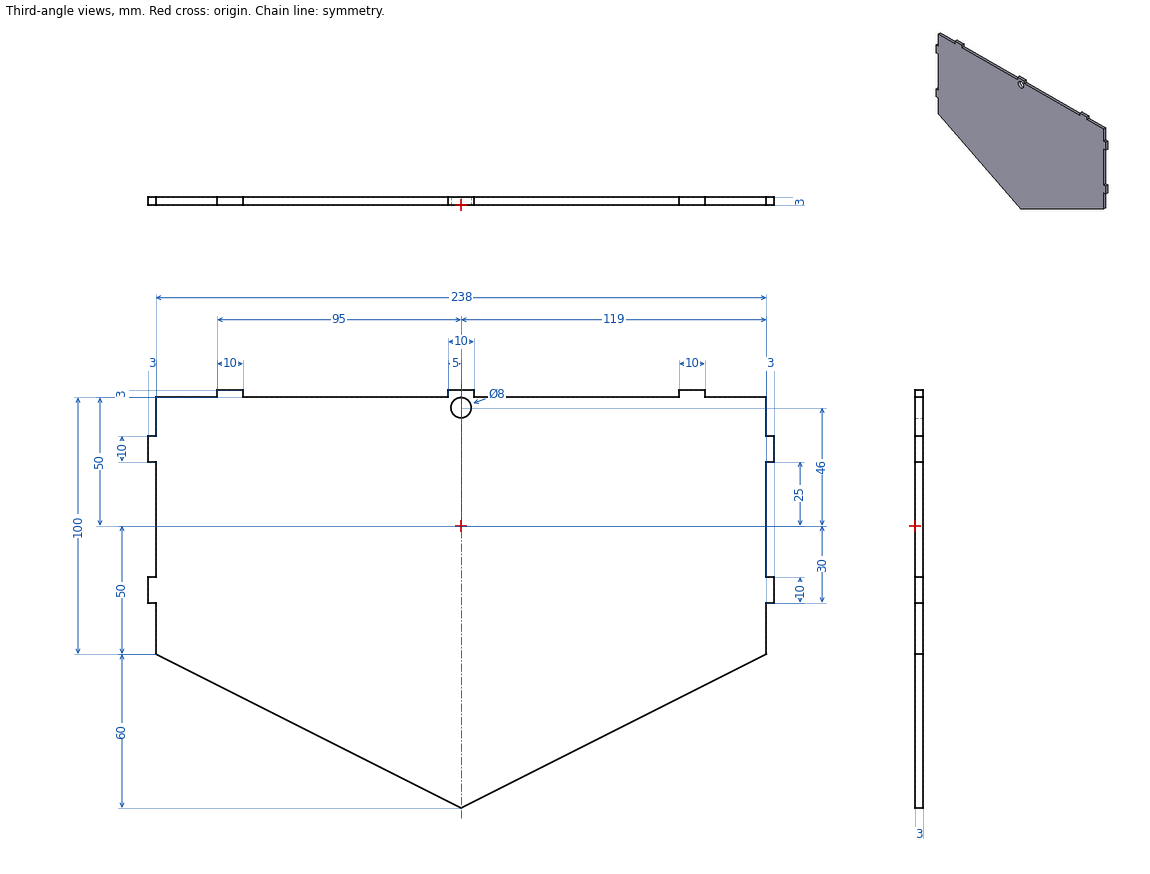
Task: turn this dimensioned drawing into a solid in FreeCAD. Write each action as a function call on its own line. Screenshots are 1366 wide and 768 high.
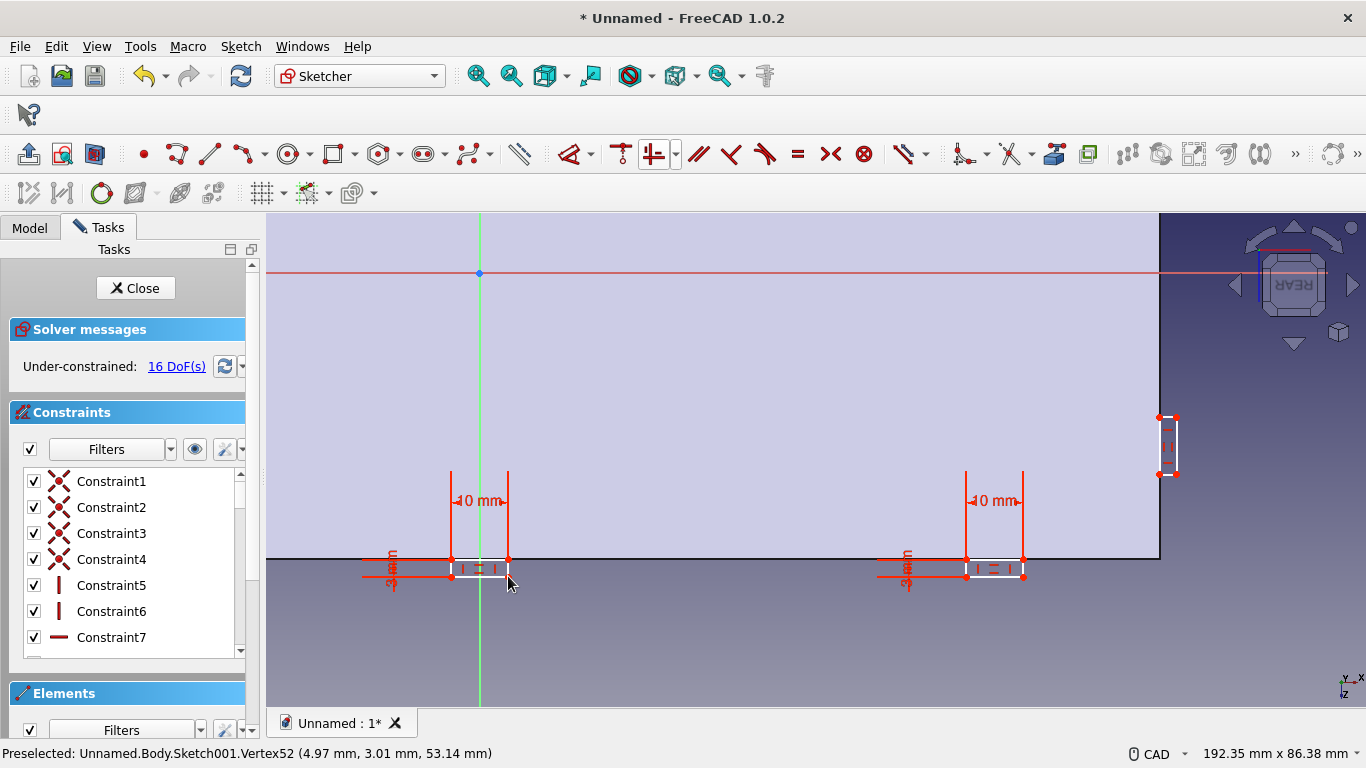
click(1177, 417)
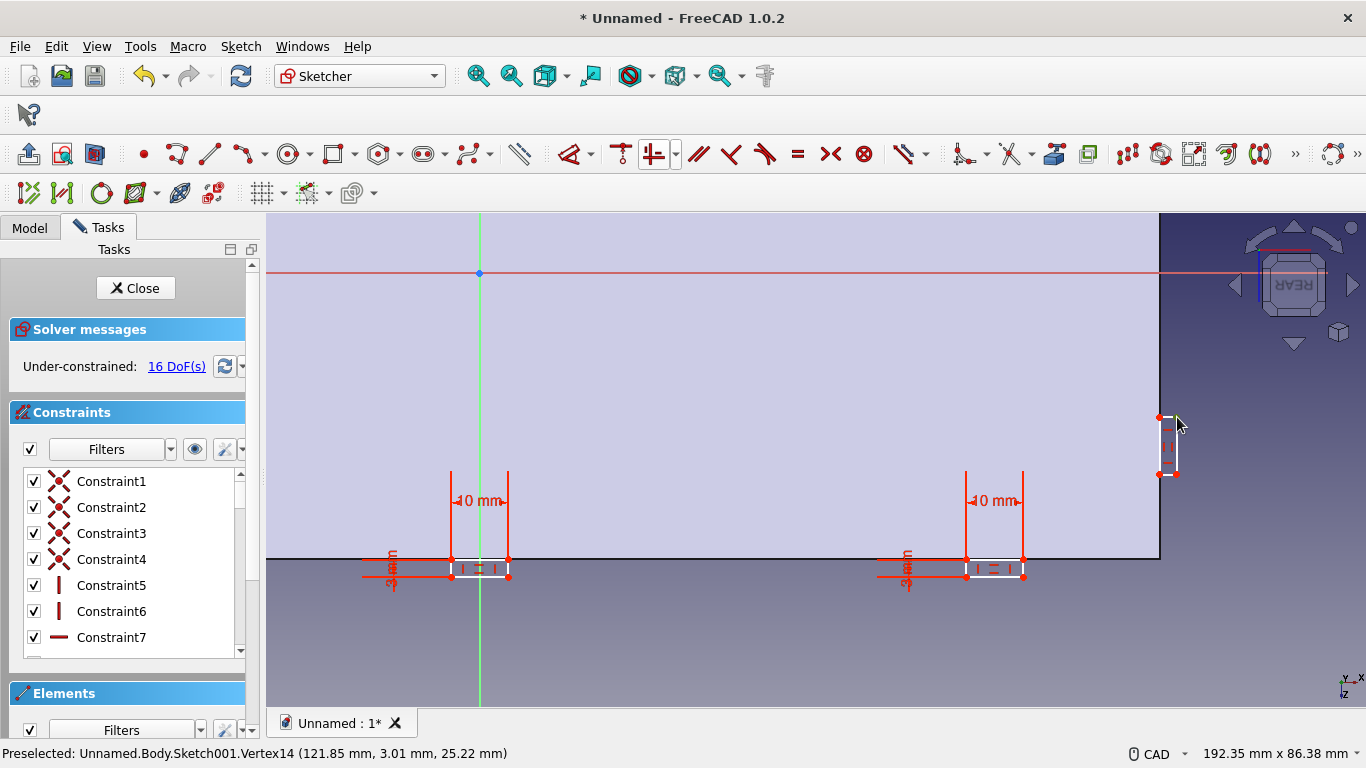
scroll(966, 559, down, 4)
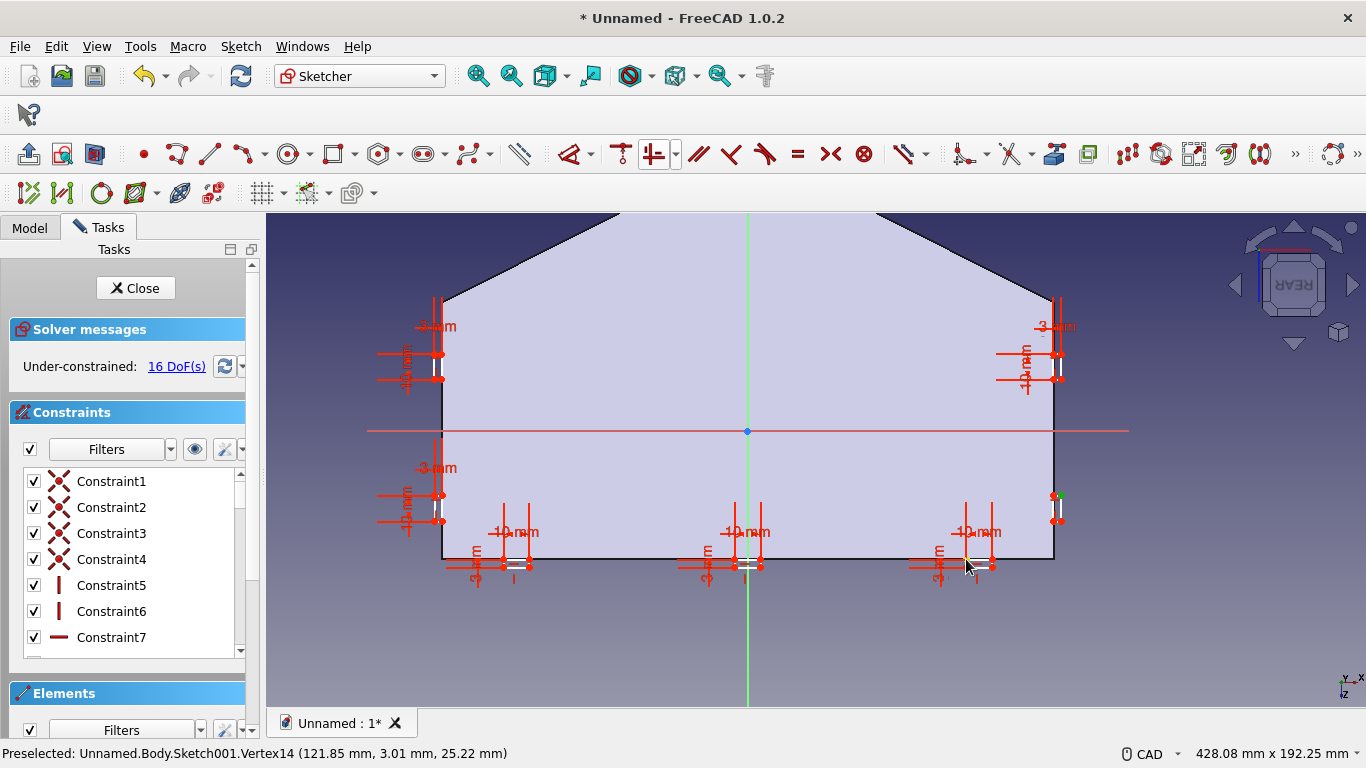
scroll(435, 496, up, 3)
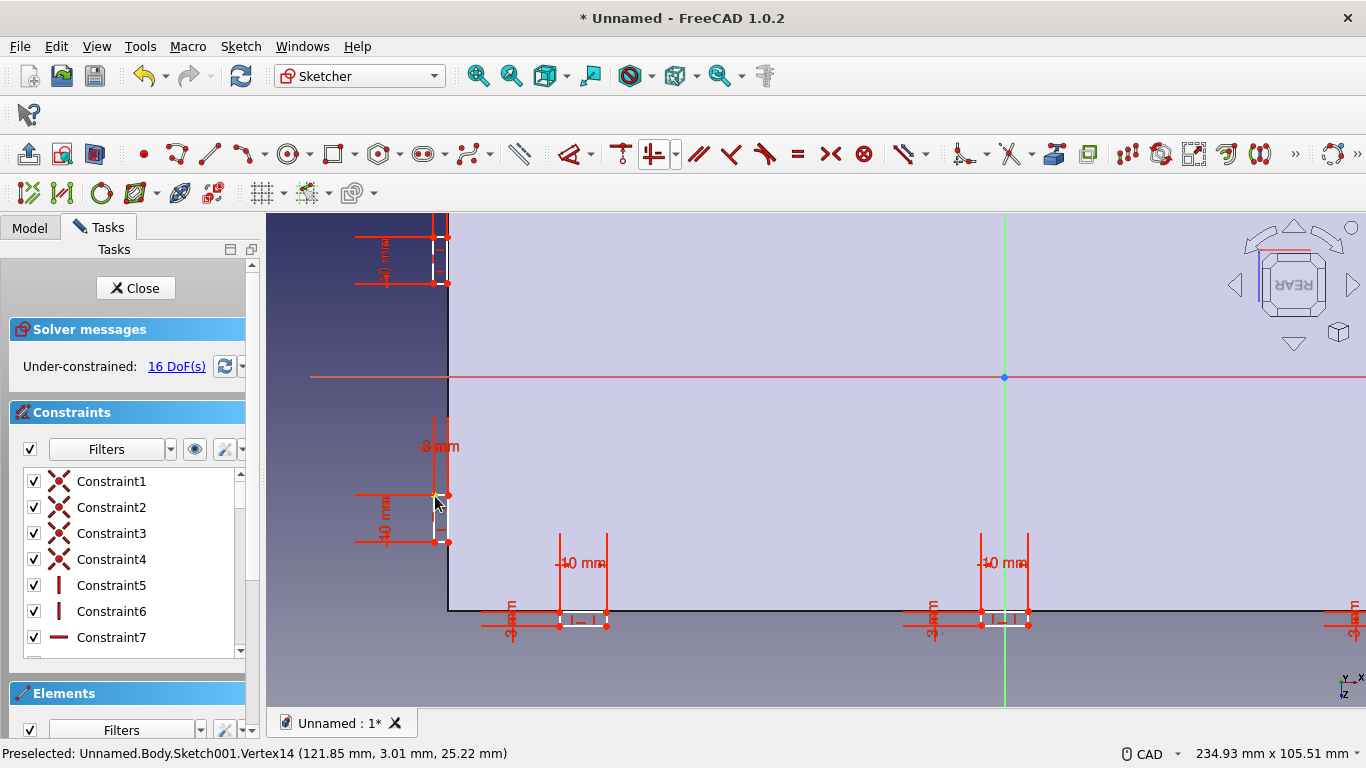
click(434, 495)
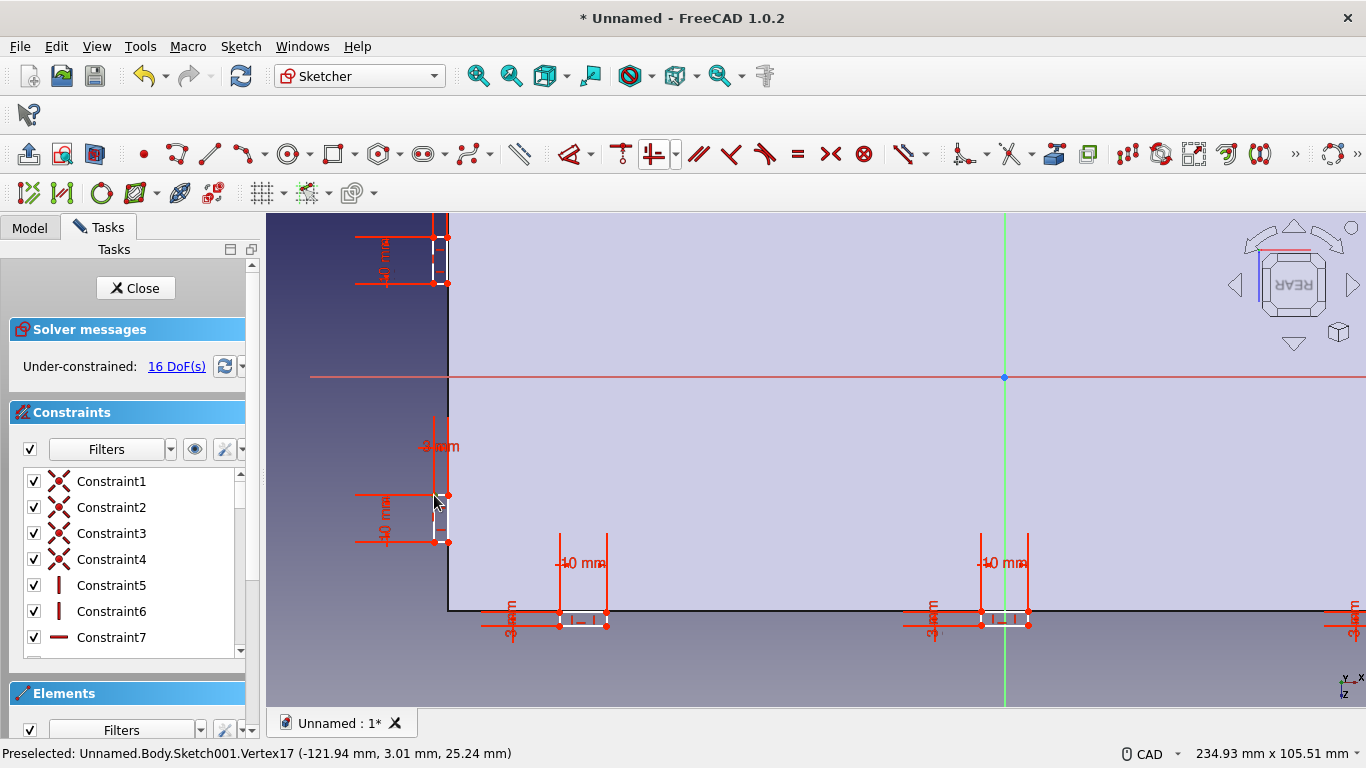
click(1005, 554)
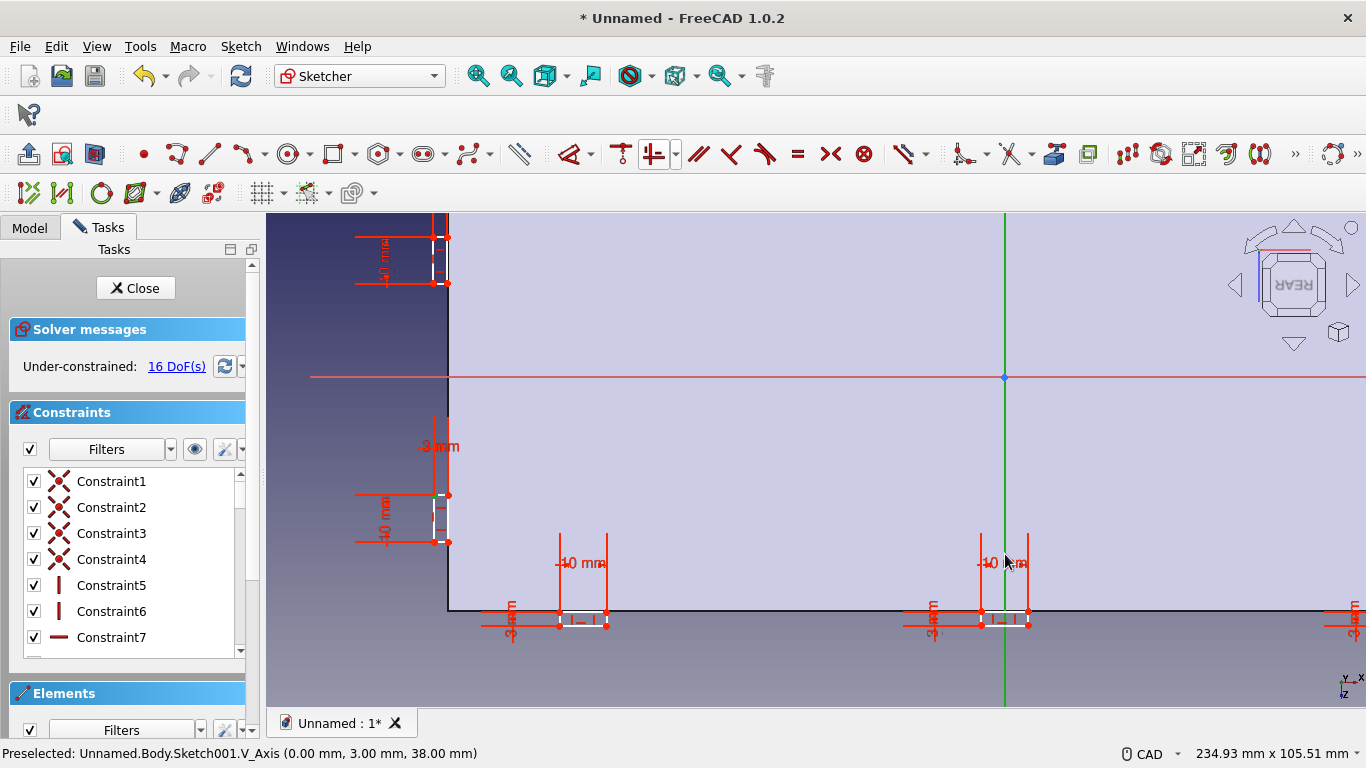
click(831, 154)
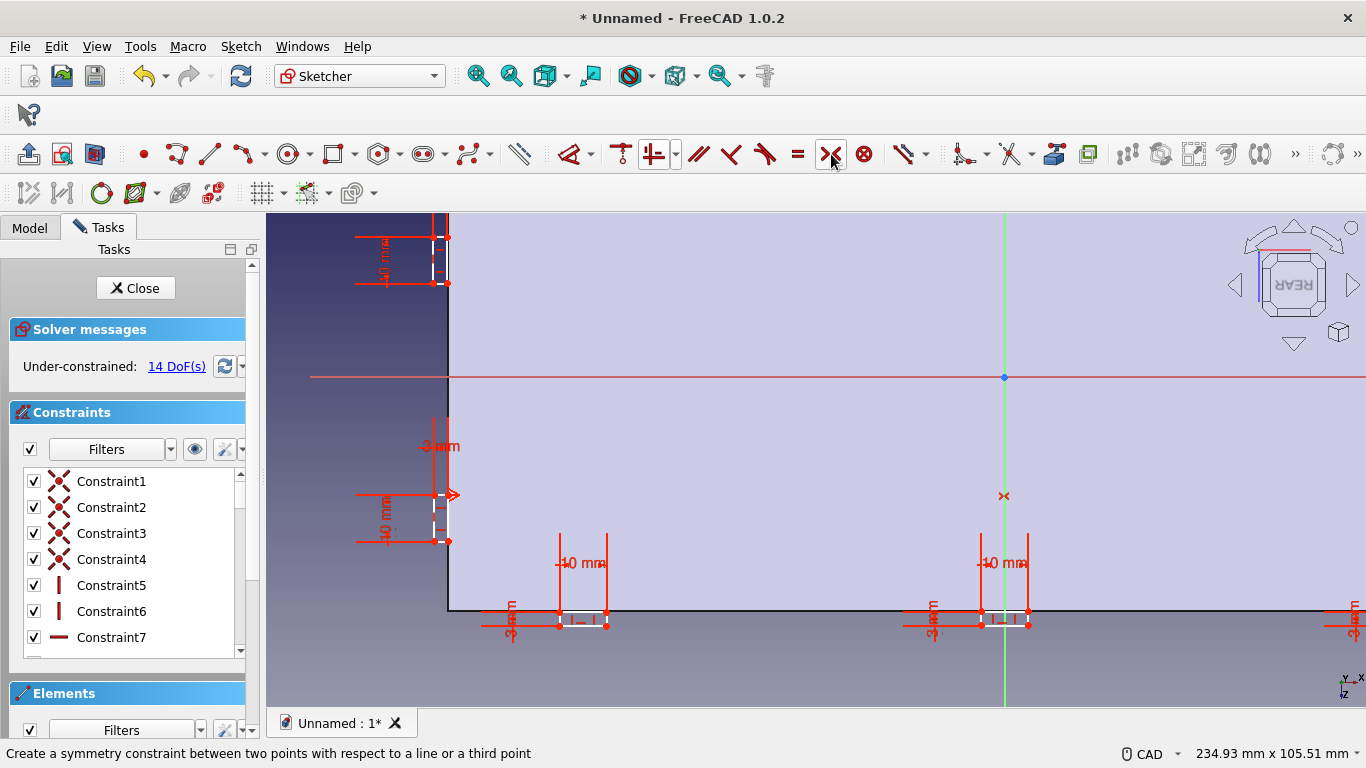
scroll(434, 495, down, 3)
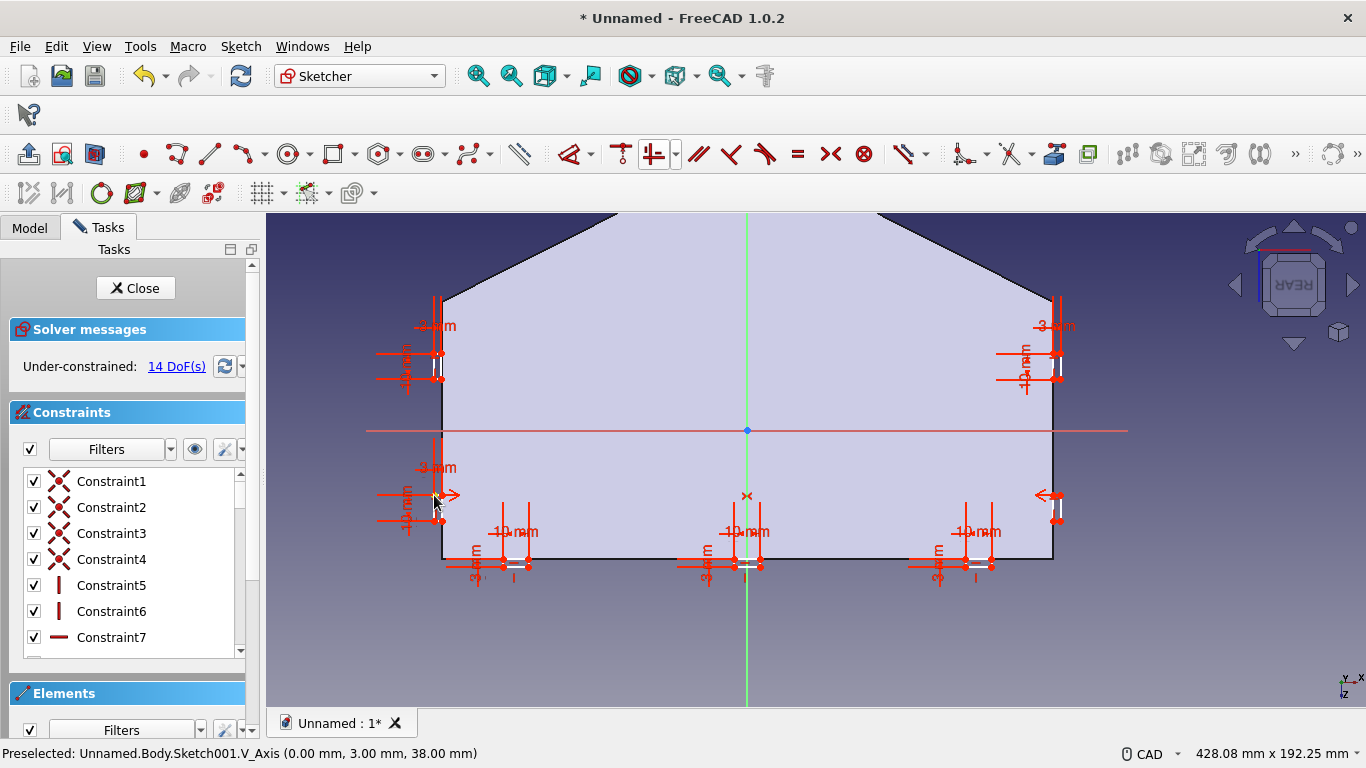
scroll(1053, 521, up, 3)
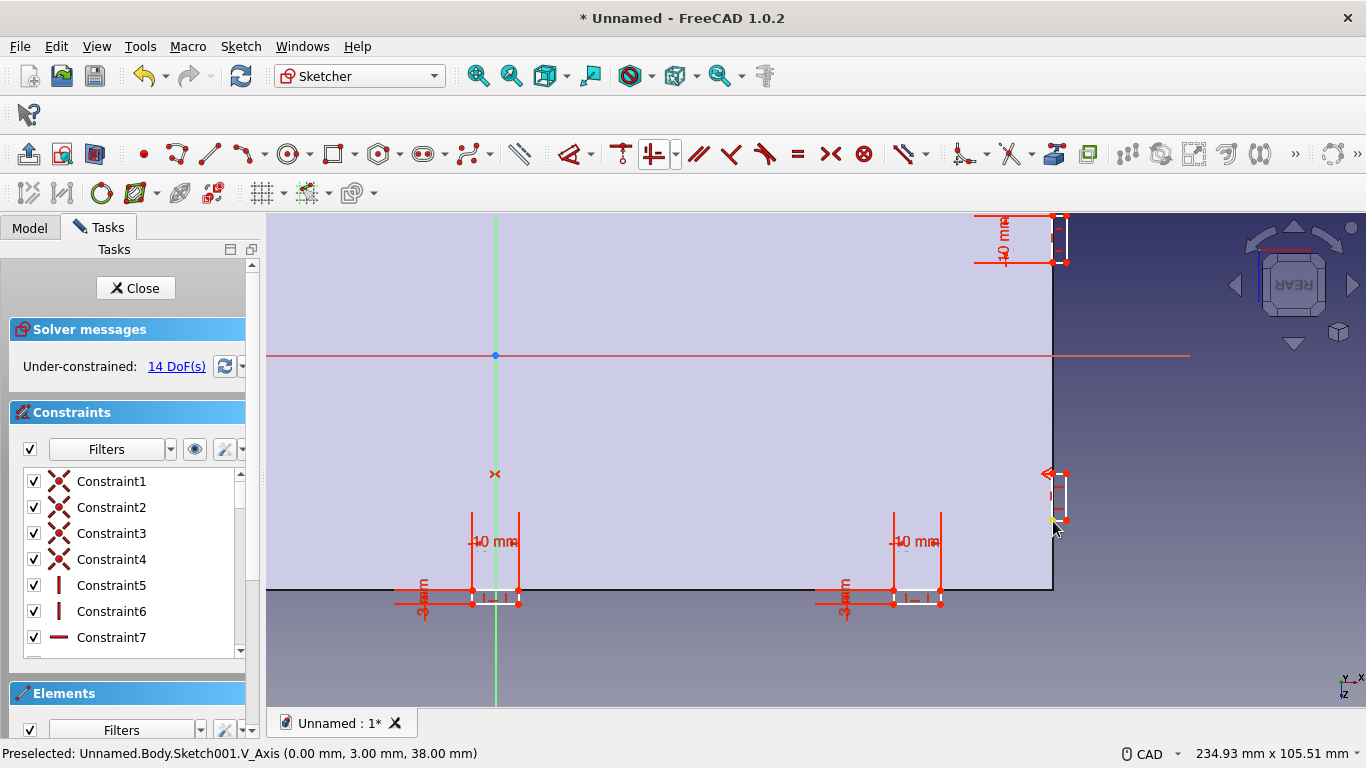
click(1052, 521)